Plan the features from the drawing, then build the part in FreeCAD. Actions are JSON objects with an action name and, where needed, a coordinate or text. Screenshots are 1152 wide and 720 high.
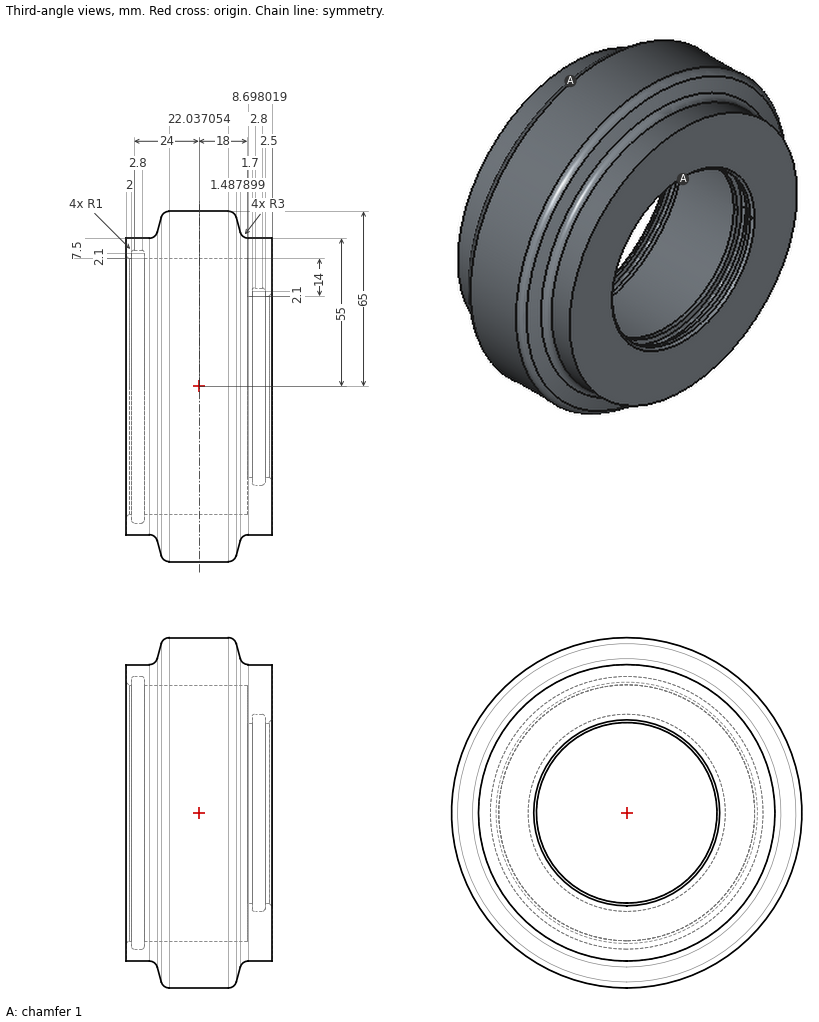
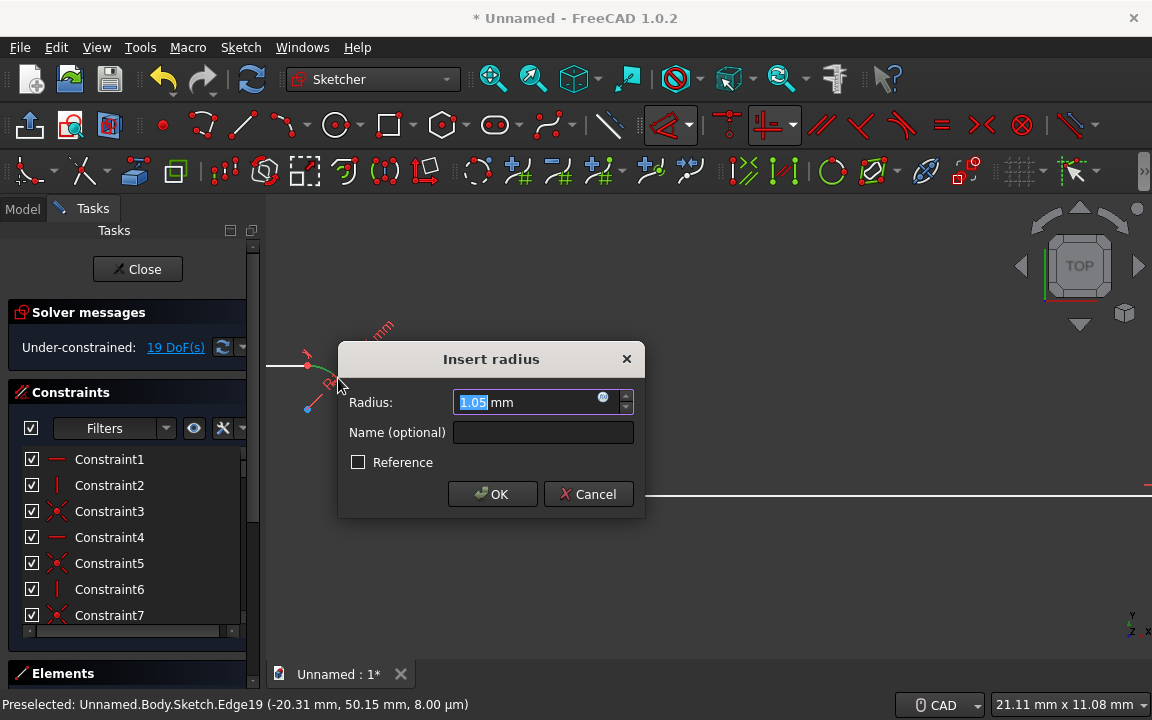
{"action": "type", "text": "1"}
{"action": "key", "text": "Return"}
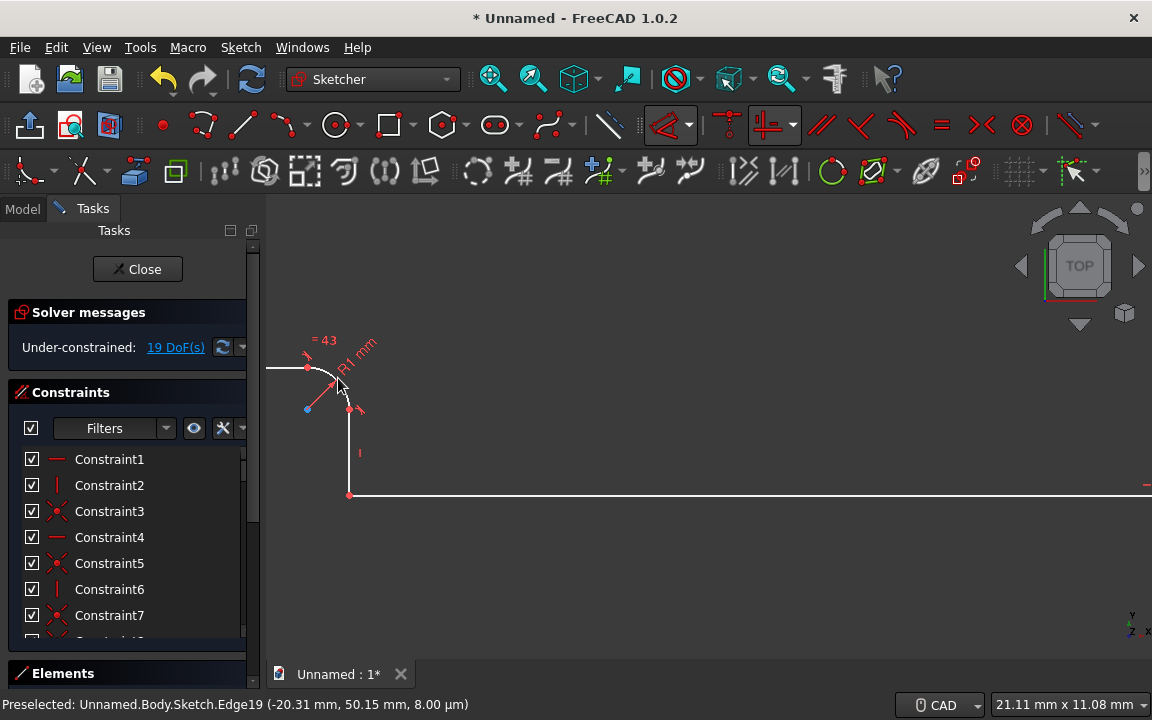
{"action": "scroll", "coordinate": [572, 340], "scroll_direction": "down", "scroll_amount": 11}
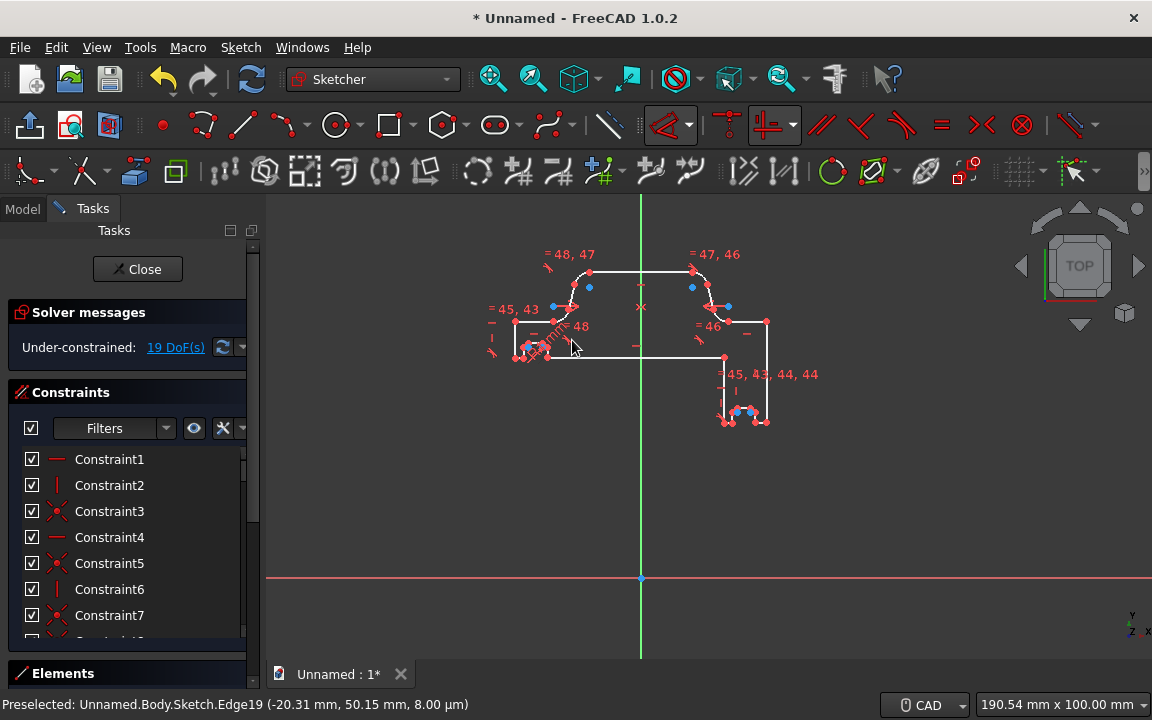
{"action": "scroll", "coordinate": [716, 316], "scroll_direction": "up", "scroll_amount": 6}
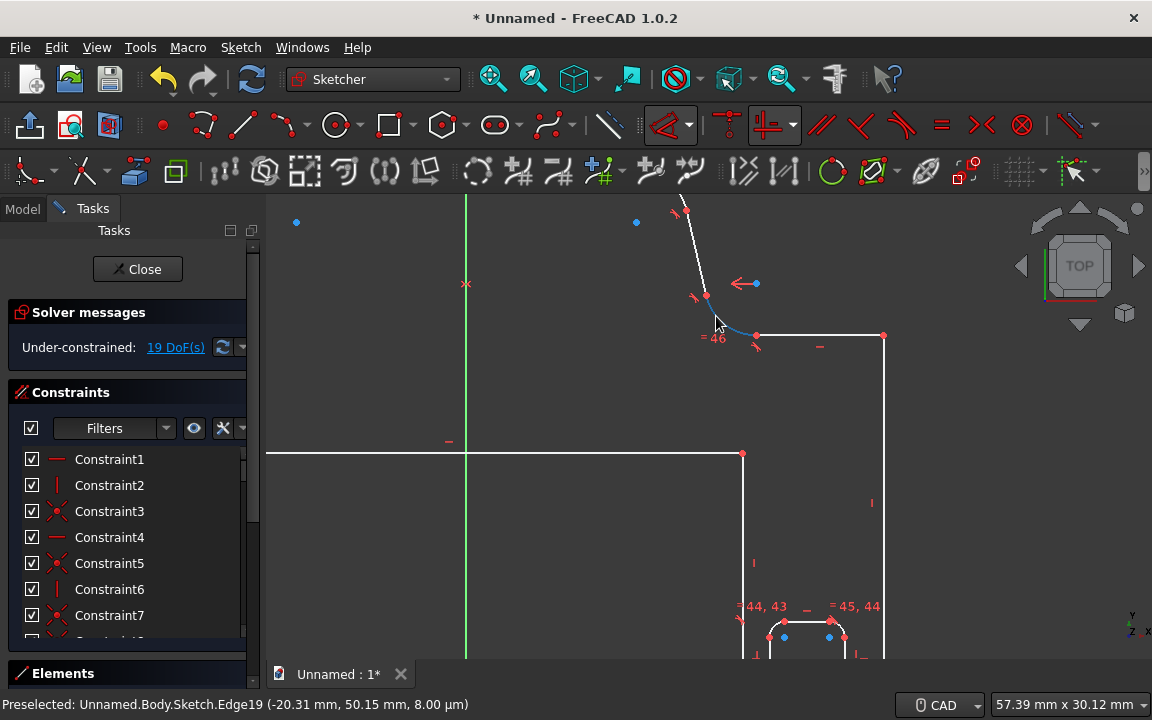
{"action": "left_click", "coordinate": [715, 314]}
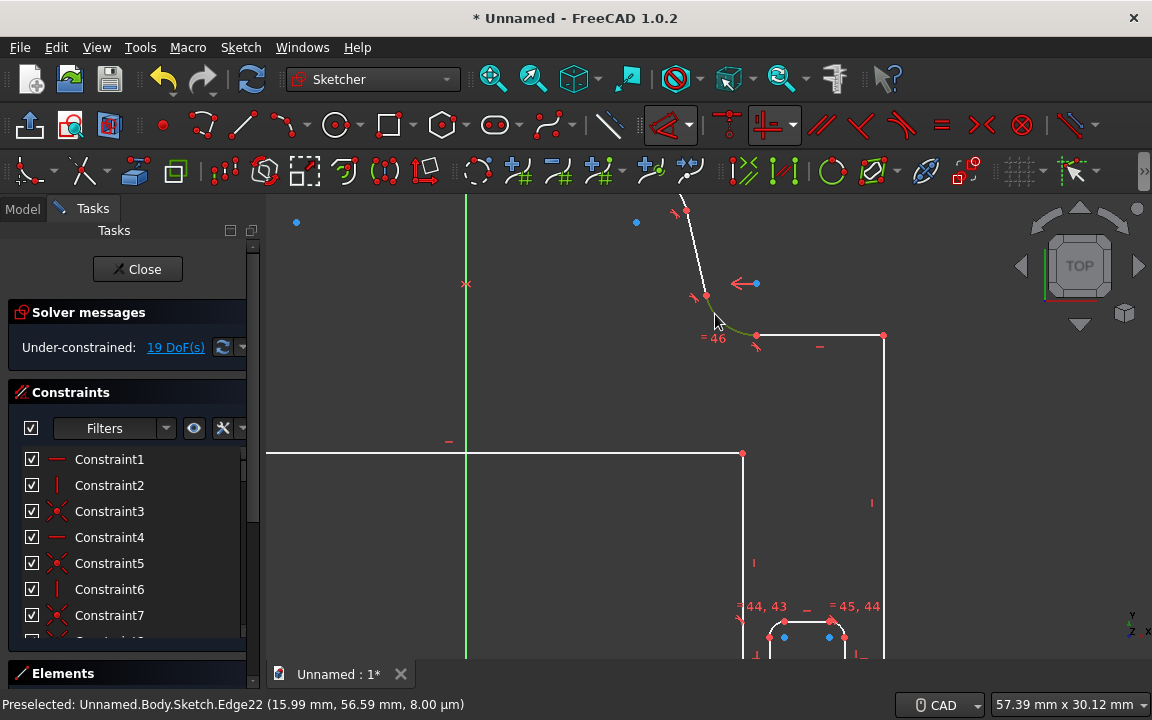
{"action": "key", "text": "k r"}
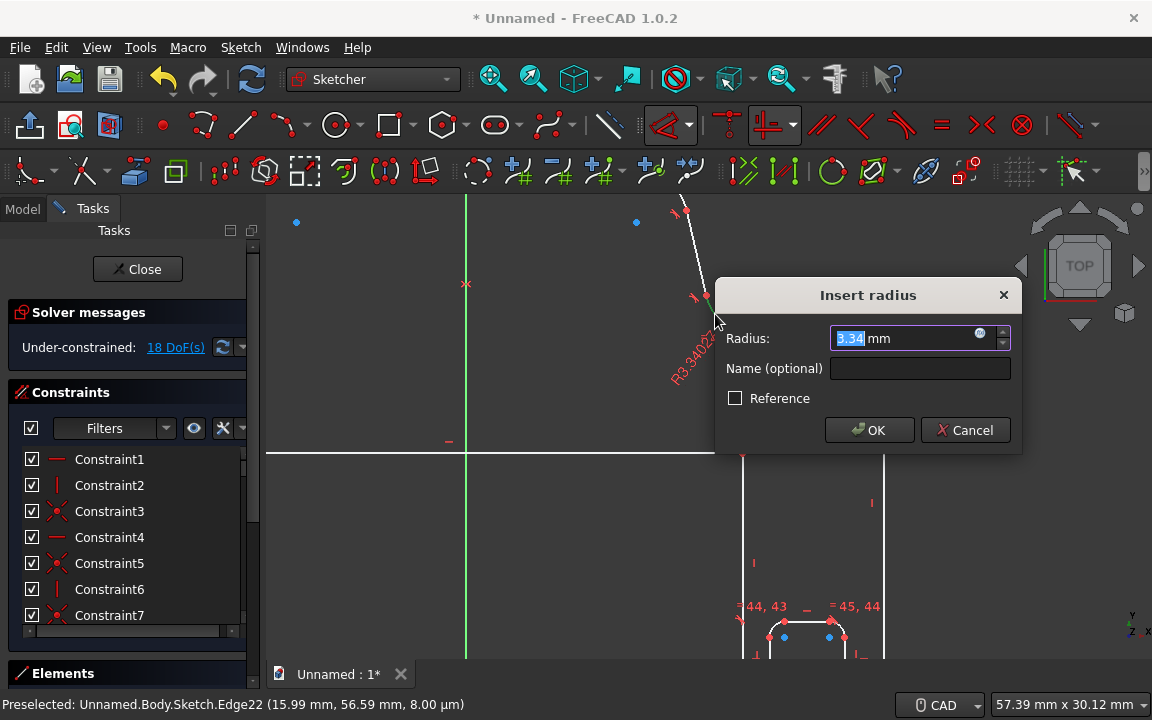
{"action": "type", "text": "3"}
{"action": "key", "text": "Return"}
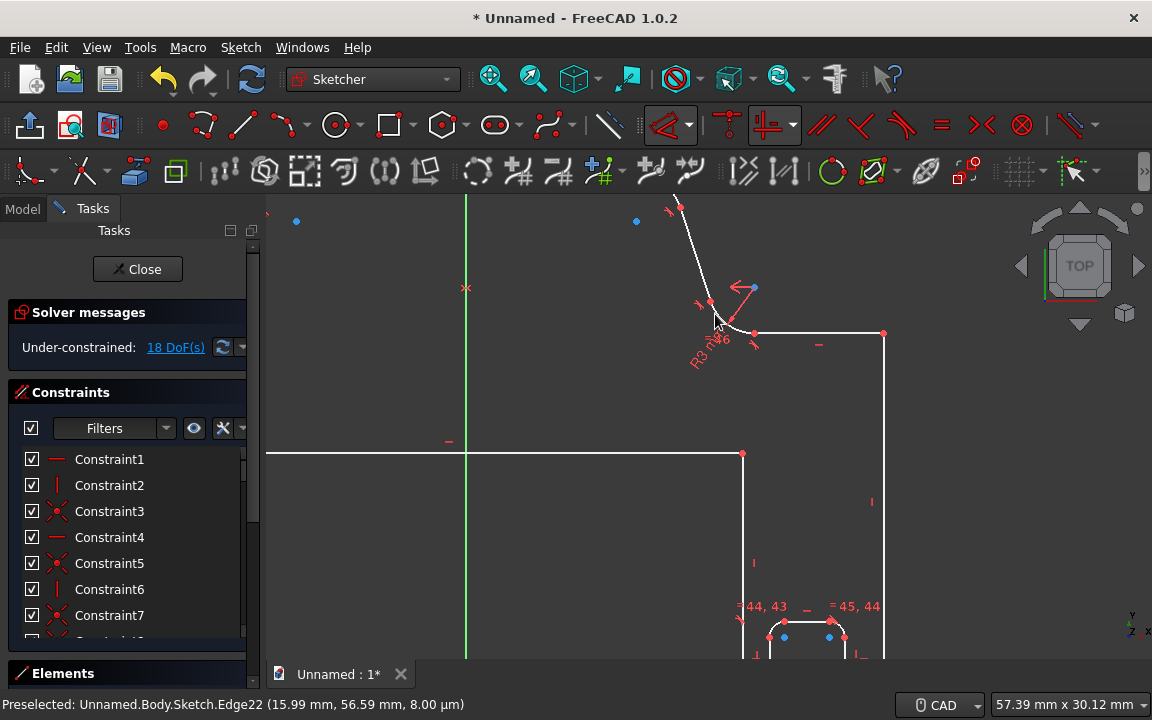
{"action": "scroll", "coordinate": [716, 316], "scroll_direction": "down", "scroll_amount": 6}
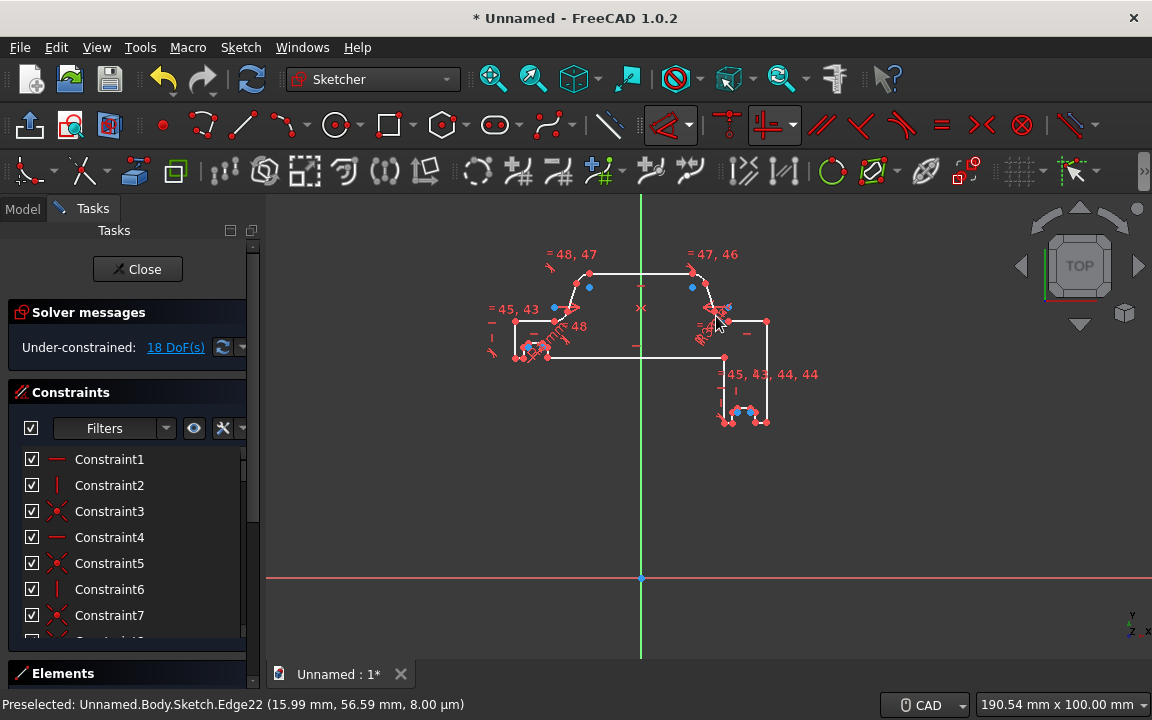
{"action": "scroll", "coordinate": [519, 358], "scroll_direction": "up", "scroll_amount": 8}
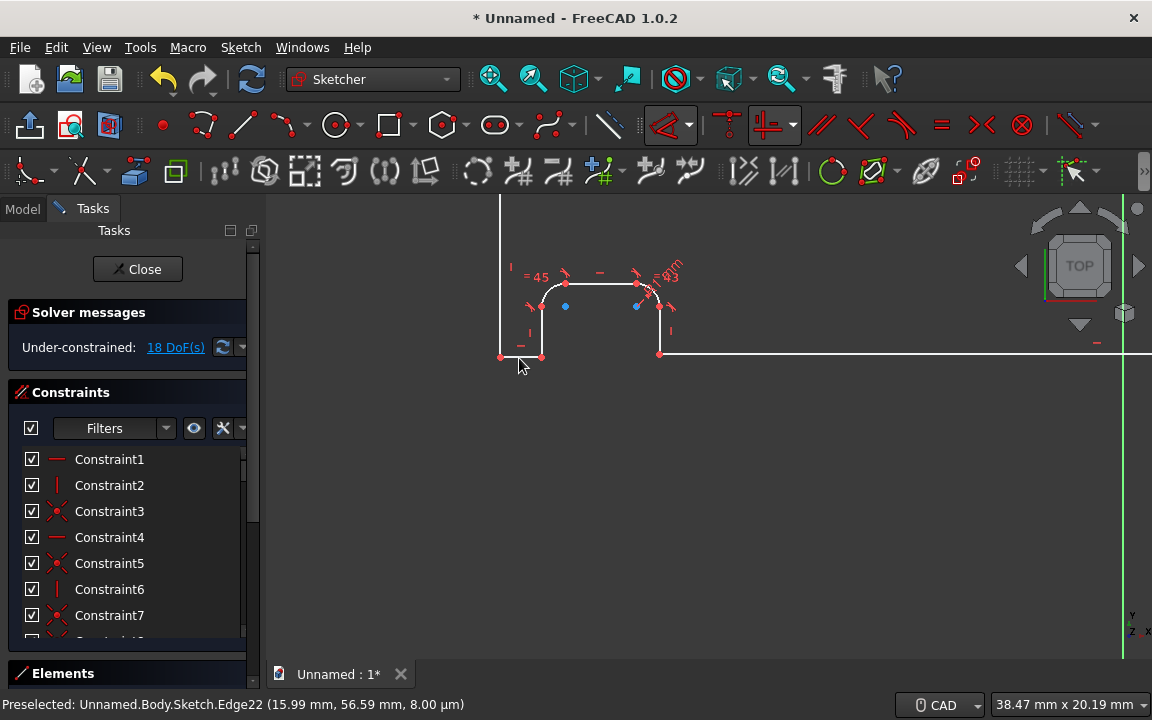
{"action": "left_click", "coordinate": [517, 357]}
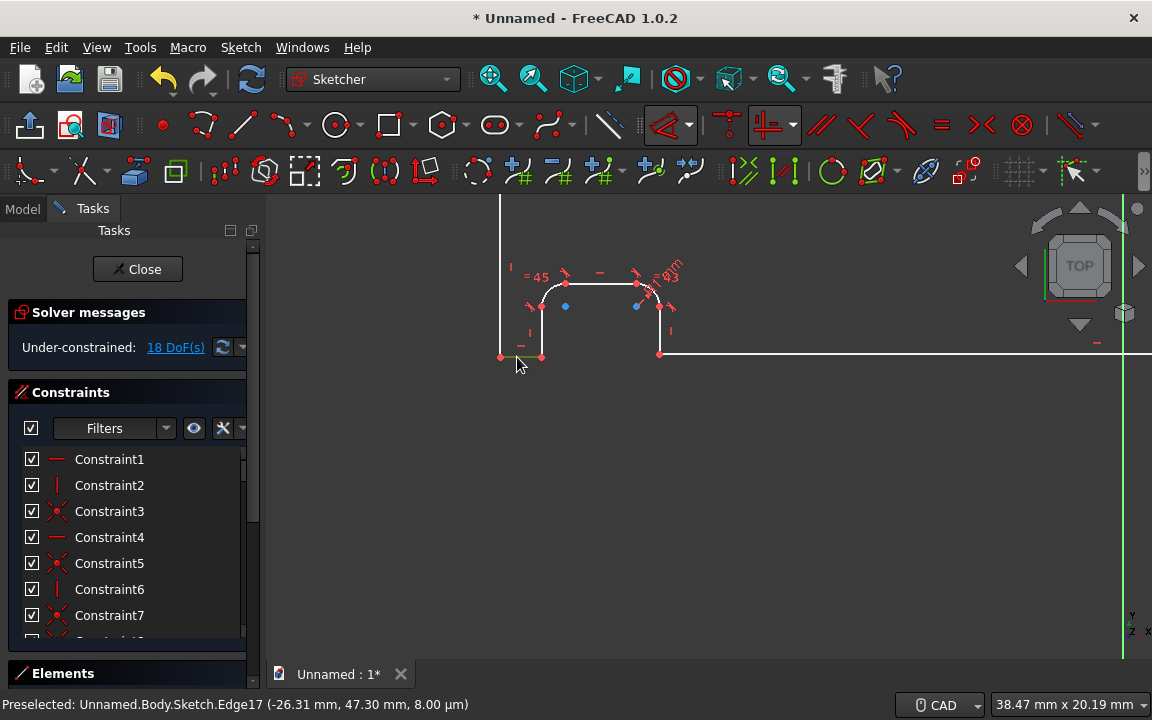
{"action": "key", "text": "l"}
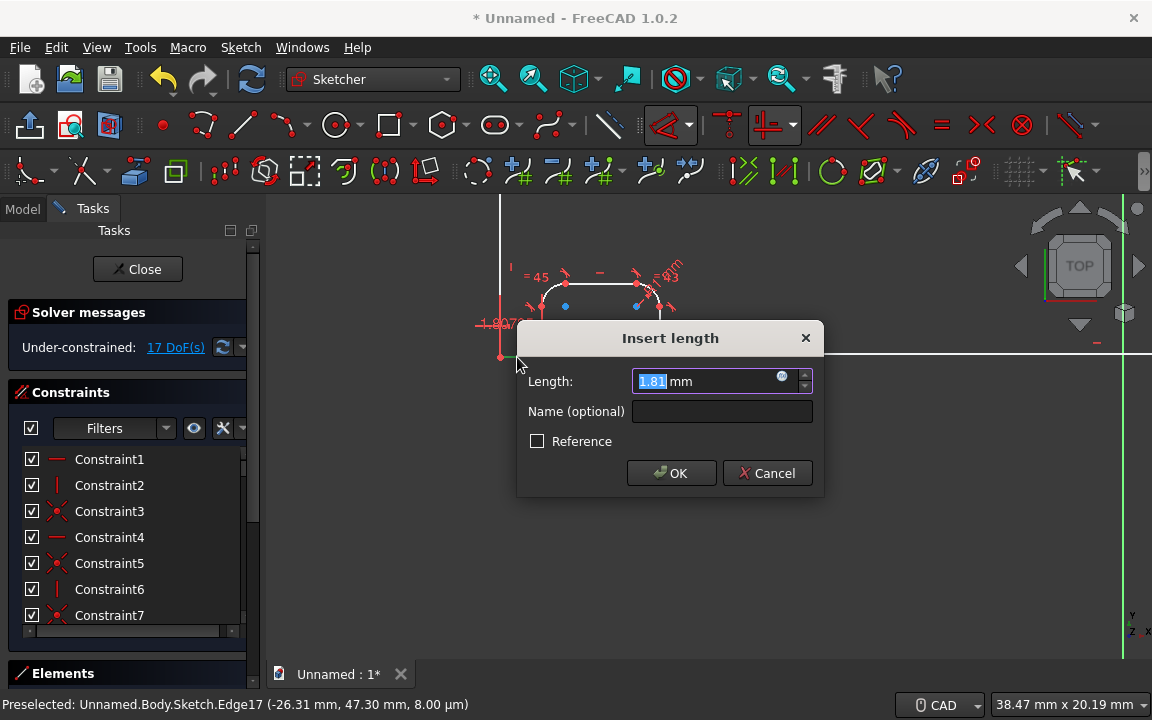
{"action": "type", "text": "2"}
{"action": "key", "text": "Return"}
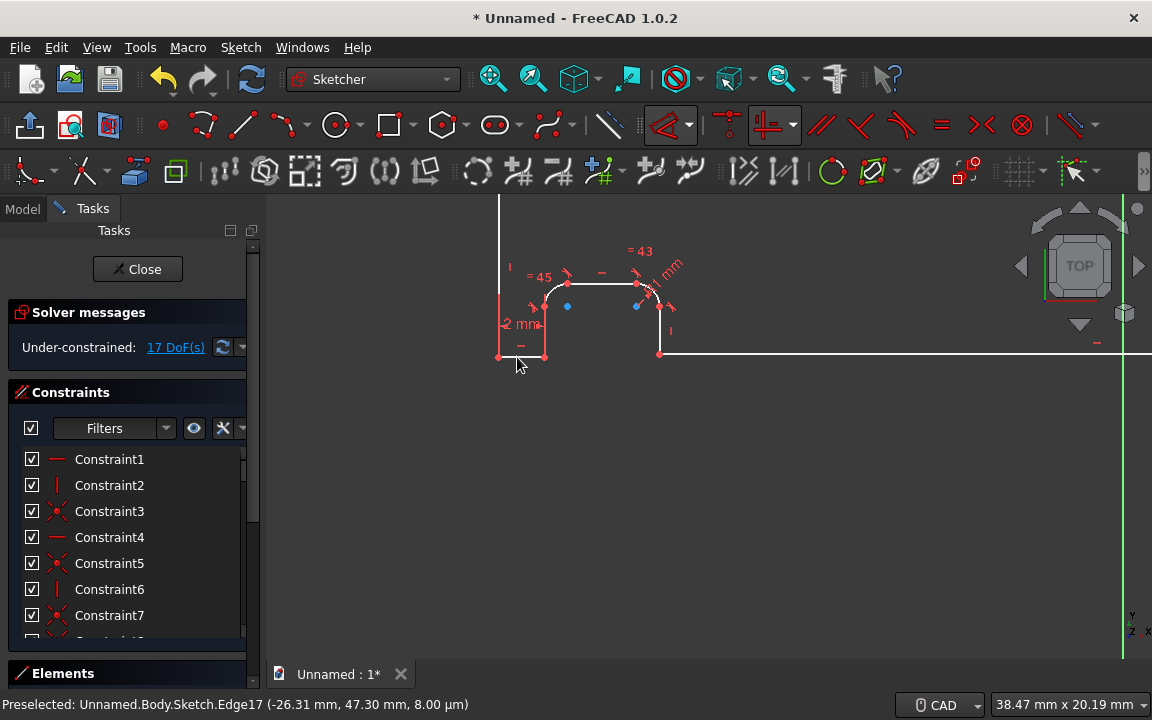
{"action": "scroll", "coordinate": [518, 358], "scroll_direction": "down", "scroll_amount": 8}